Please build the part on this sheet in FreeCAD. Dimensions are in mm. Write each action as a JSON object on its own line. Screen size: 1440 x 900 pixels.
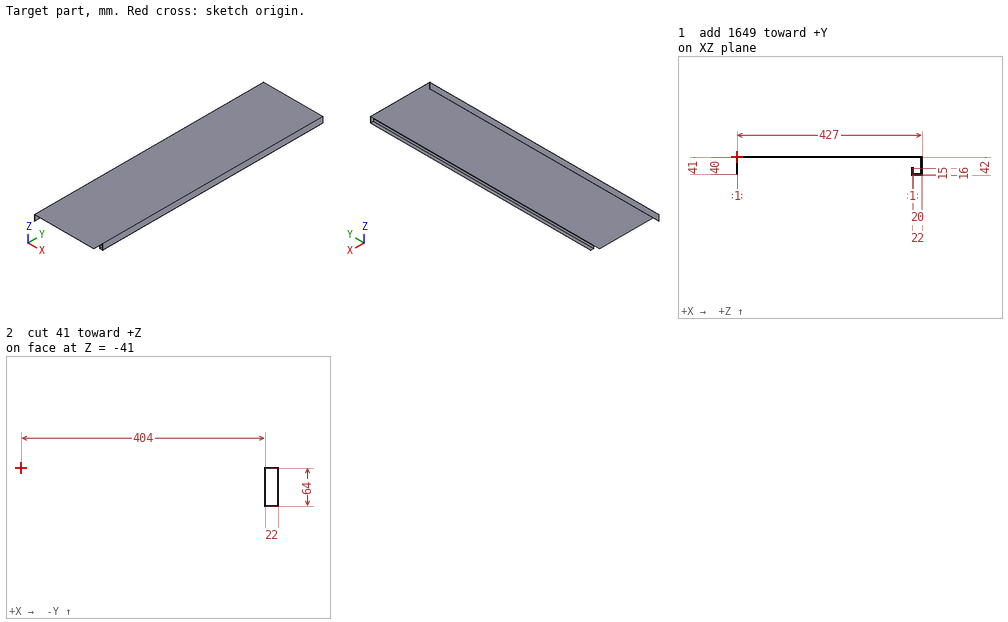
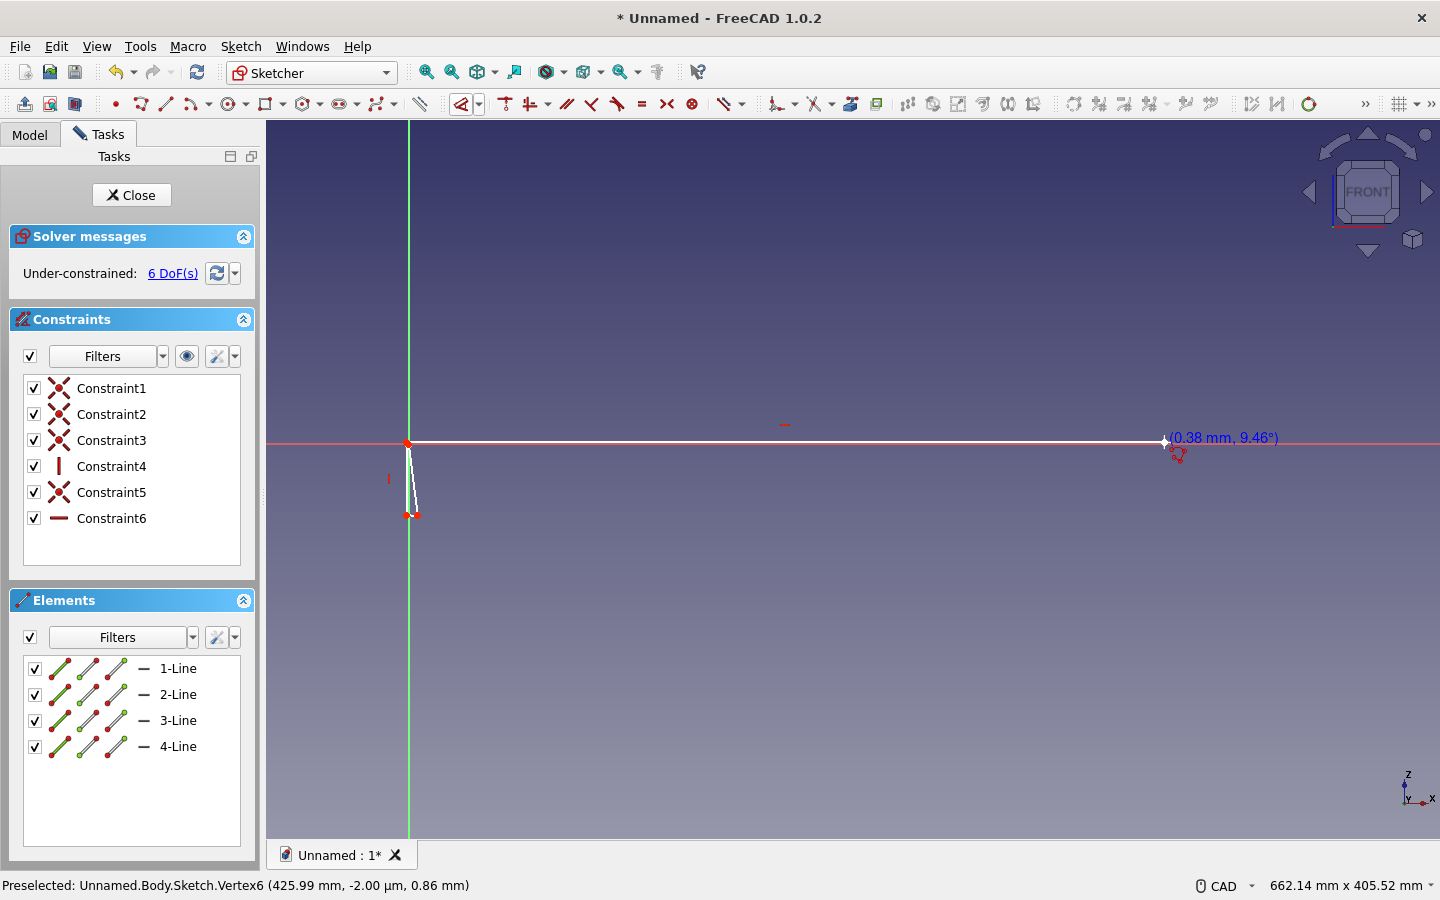
{"action": "left_click", "coordinate": [1164, 517]}
{"action": "left_click", "coordinate": [1125, 517]}
{"action": "left_click", "coordinate": [1125, 488]}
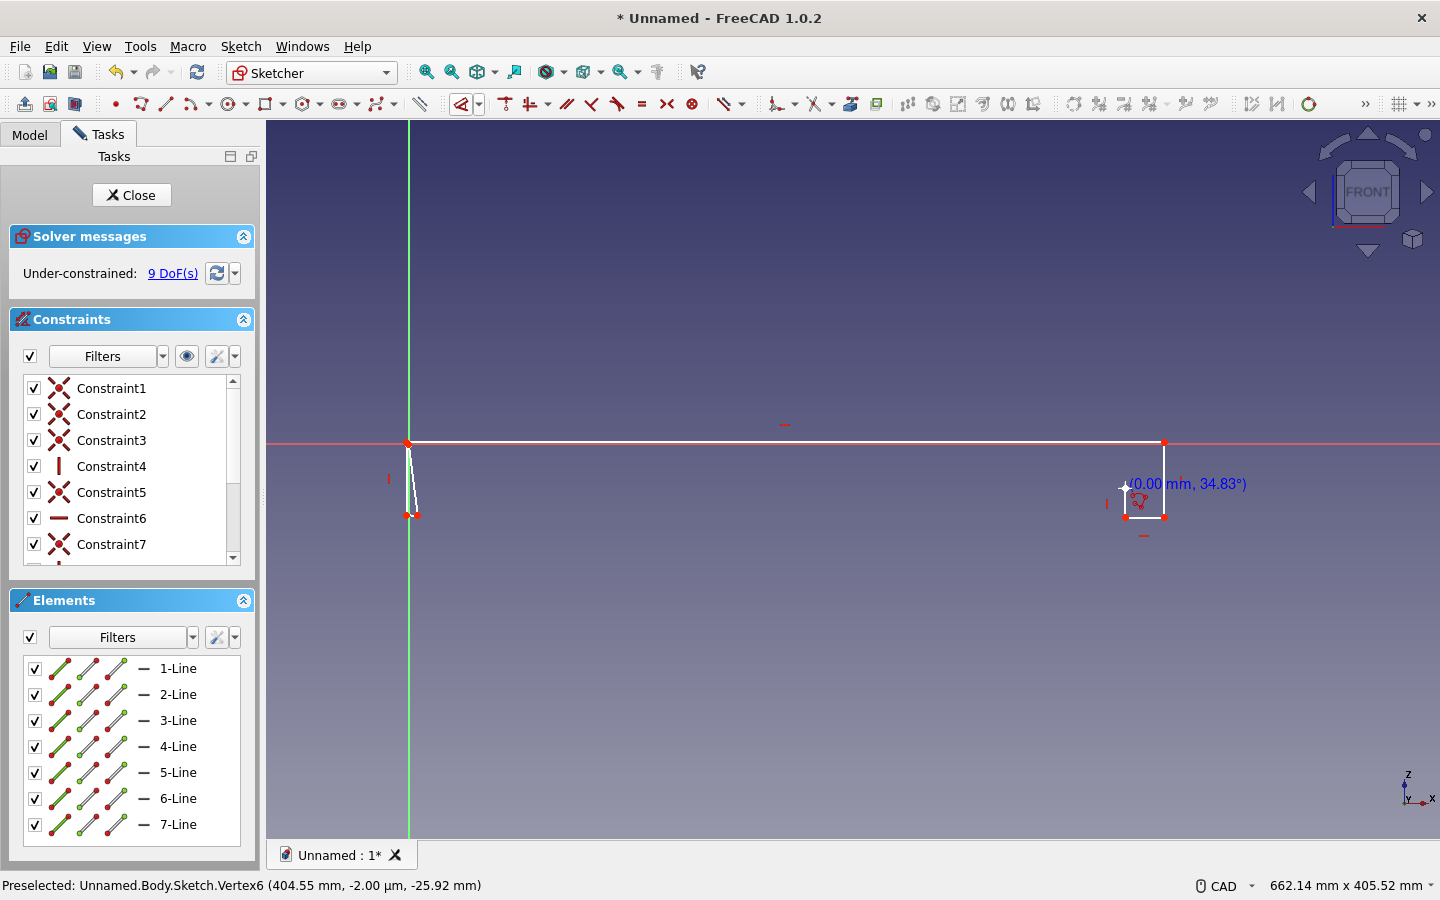
{"action": "scroll", "coordinate": [1127, 488], "scroll_direction": "up", "scroll_amount": 11}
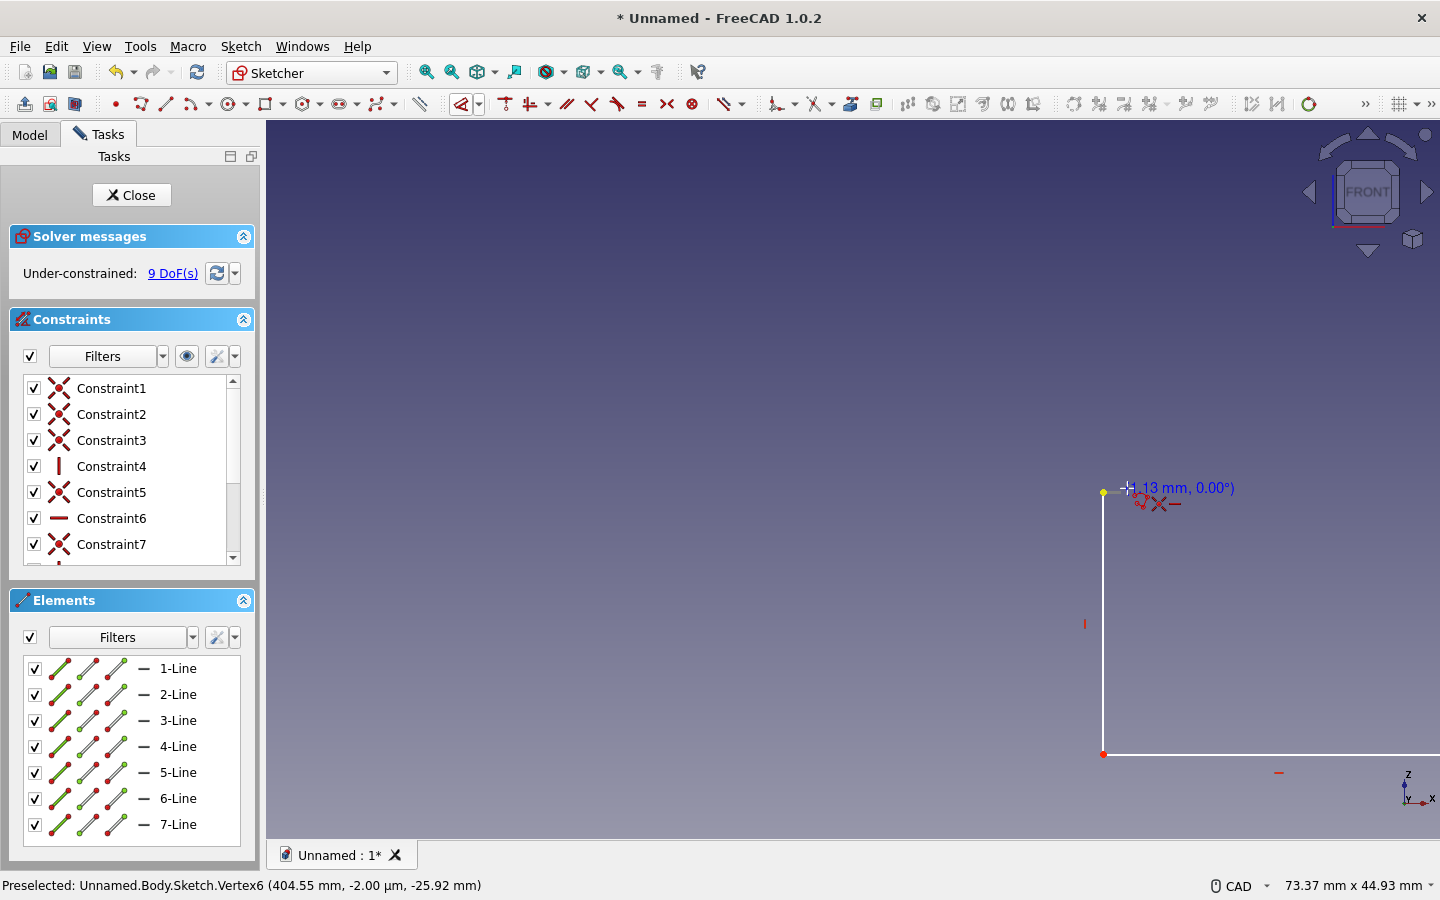
{"action": "left_click", "coordinate": [1119, 484]}
{"action": "left_click", "coordinate": [1119, 727]}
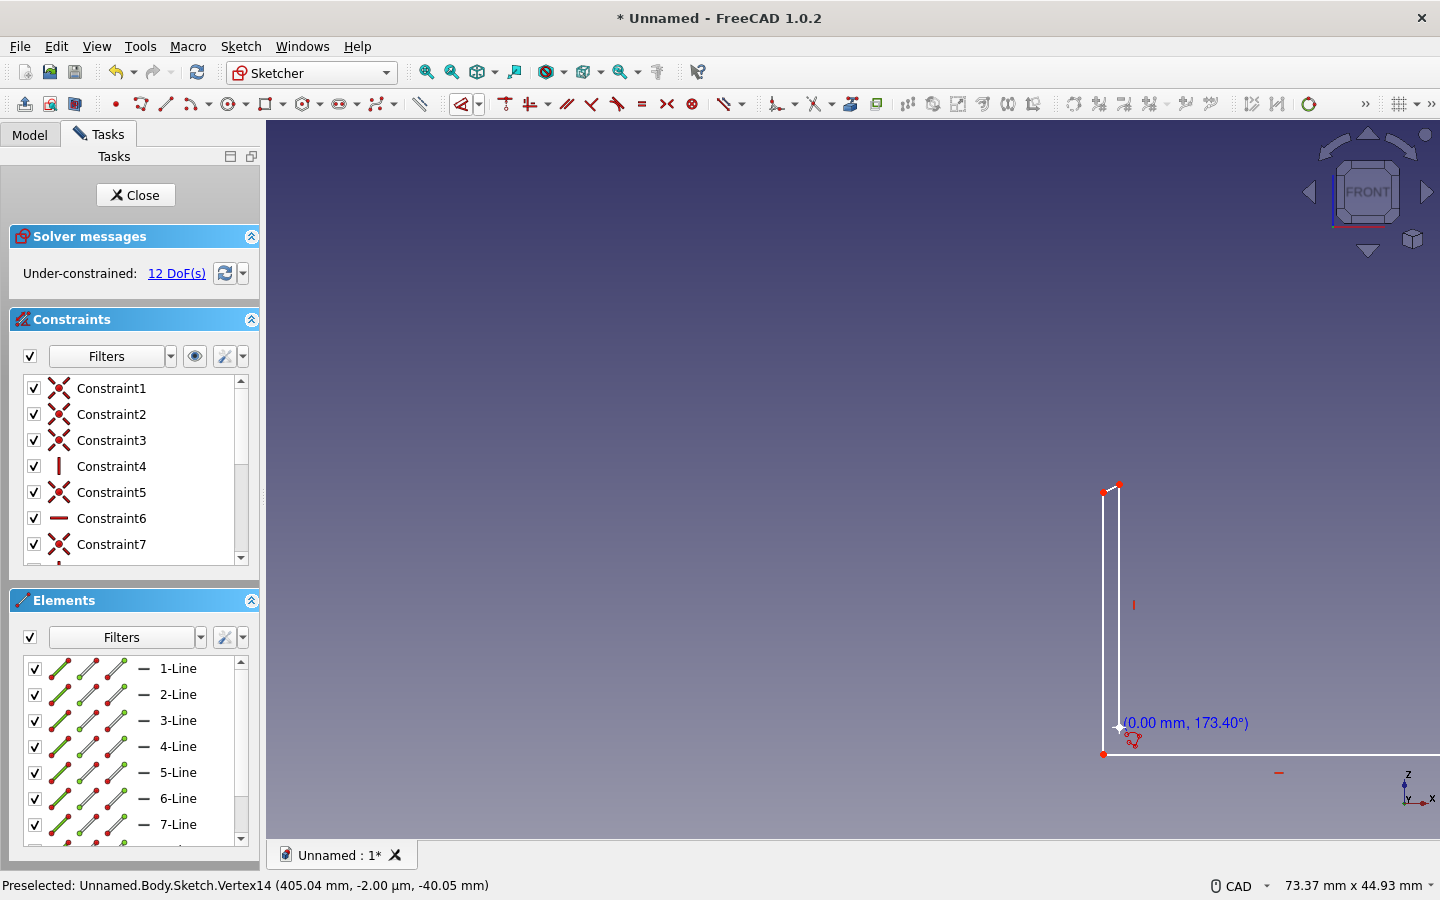
{"action": "scroll", "coordinate": [1127, 489], "scroll_direction": "down", "scroll_amount": 11}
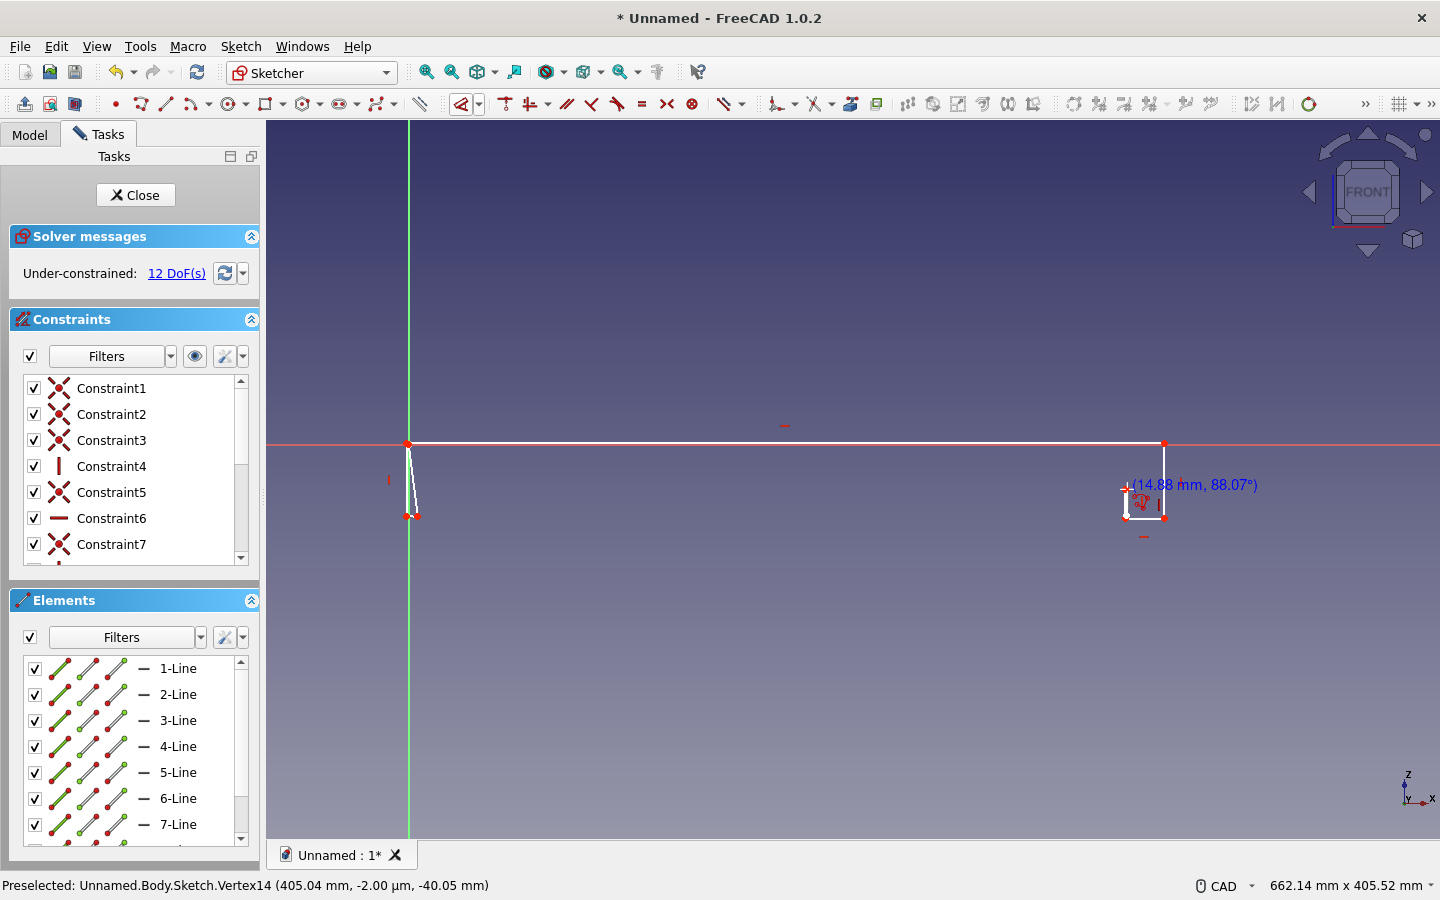
{"action": "scroll", "coordinate": [1162, 516], "scroll_direction": "up", "scroll_amount": 11}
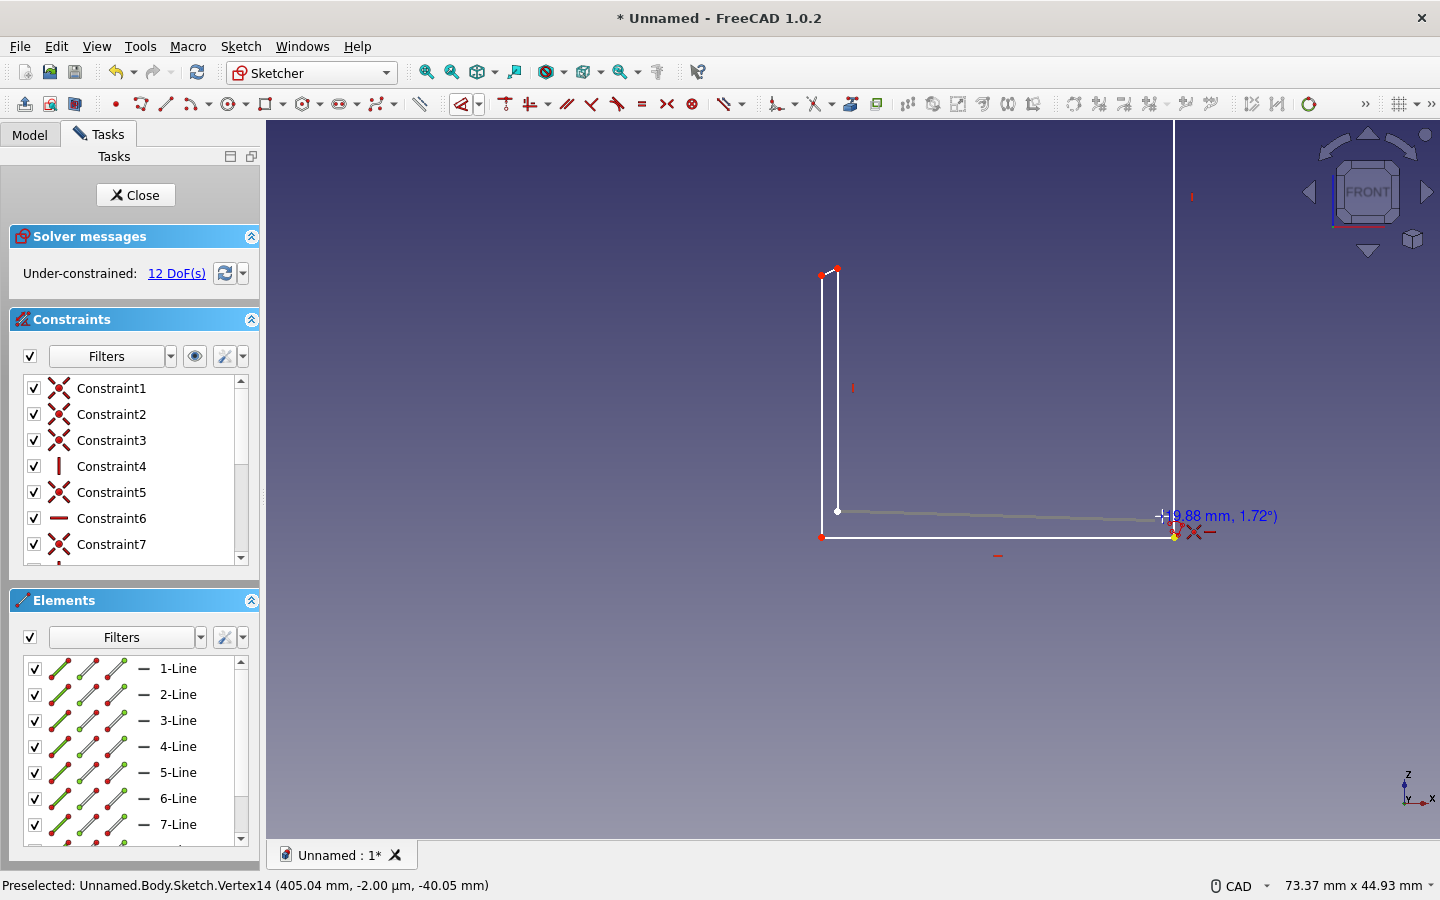
{"action": "left_click", "coordinate": [1158, 510]}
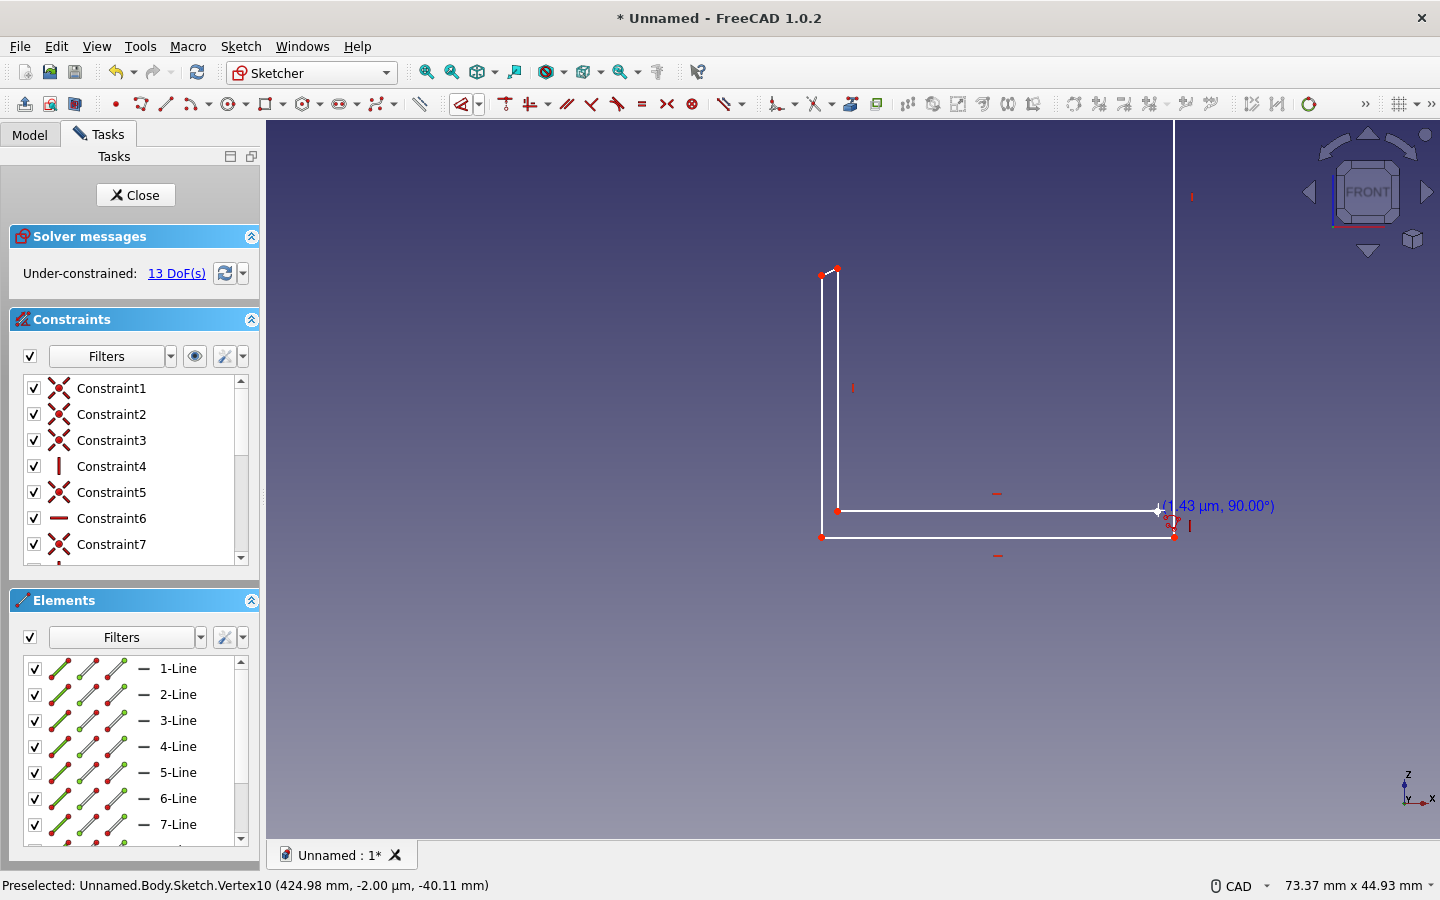
{"action": "scroll", "coordinate": [1162, 516], "scroll_direction": "down", "scroll_amount": 11}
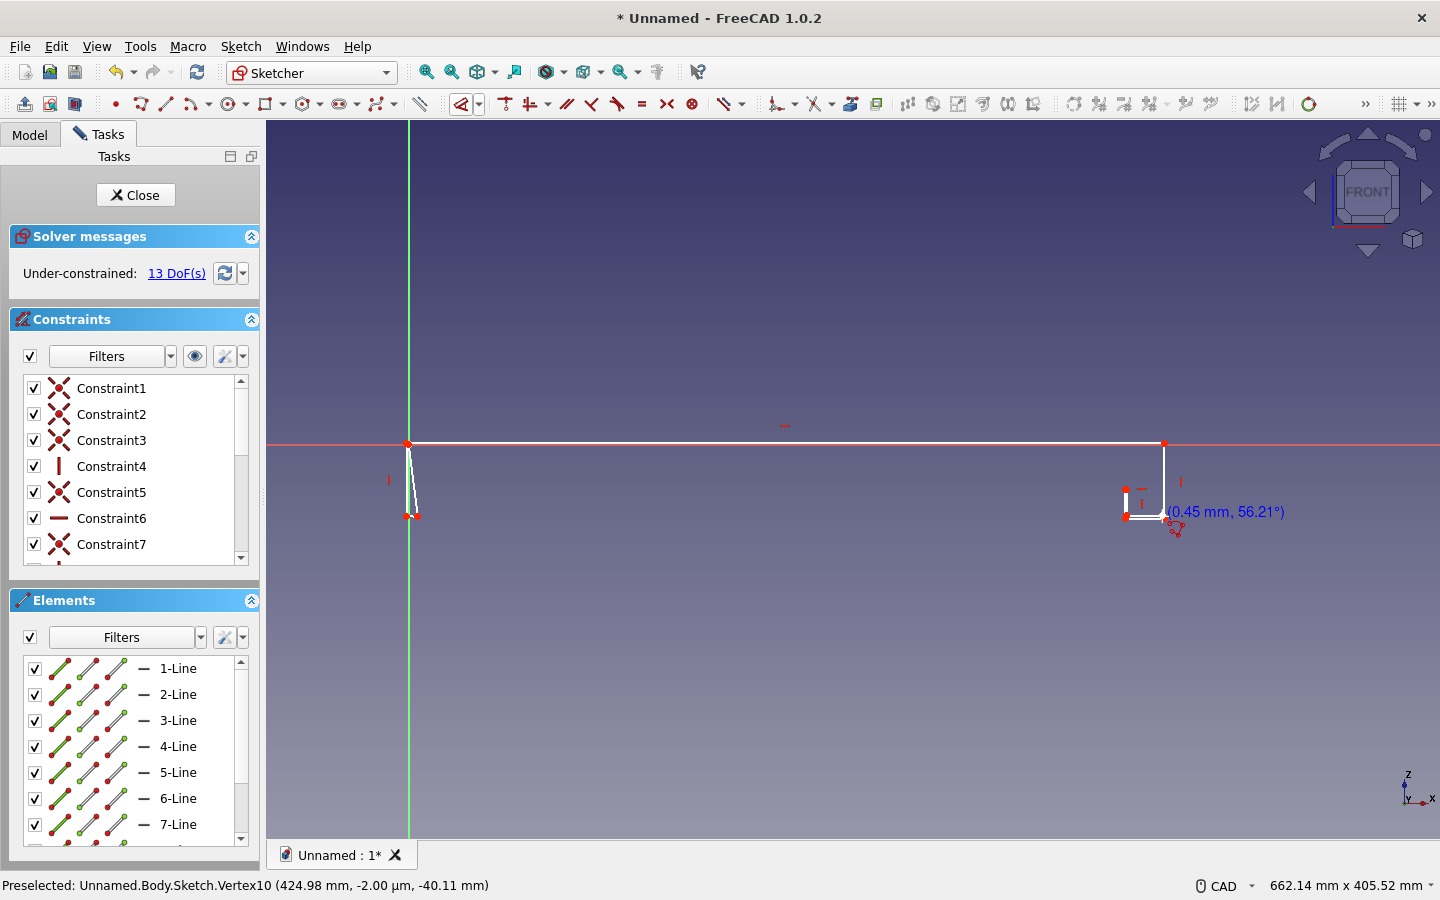
{"action": "scroll", "coordinate": [1162, 445], "scroll_direction": "up", "scroll_amount": 11}